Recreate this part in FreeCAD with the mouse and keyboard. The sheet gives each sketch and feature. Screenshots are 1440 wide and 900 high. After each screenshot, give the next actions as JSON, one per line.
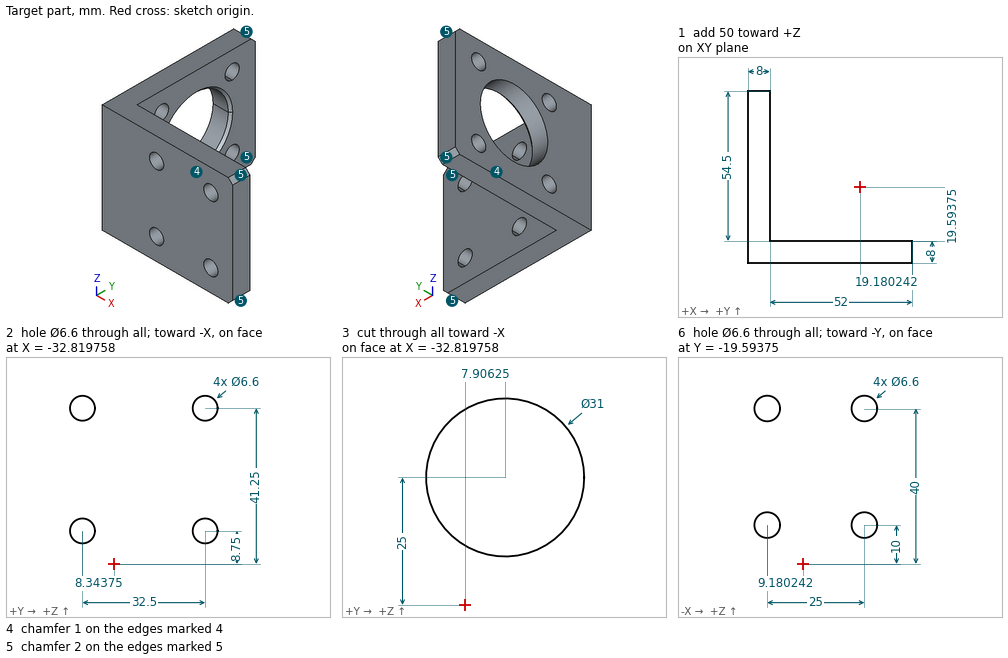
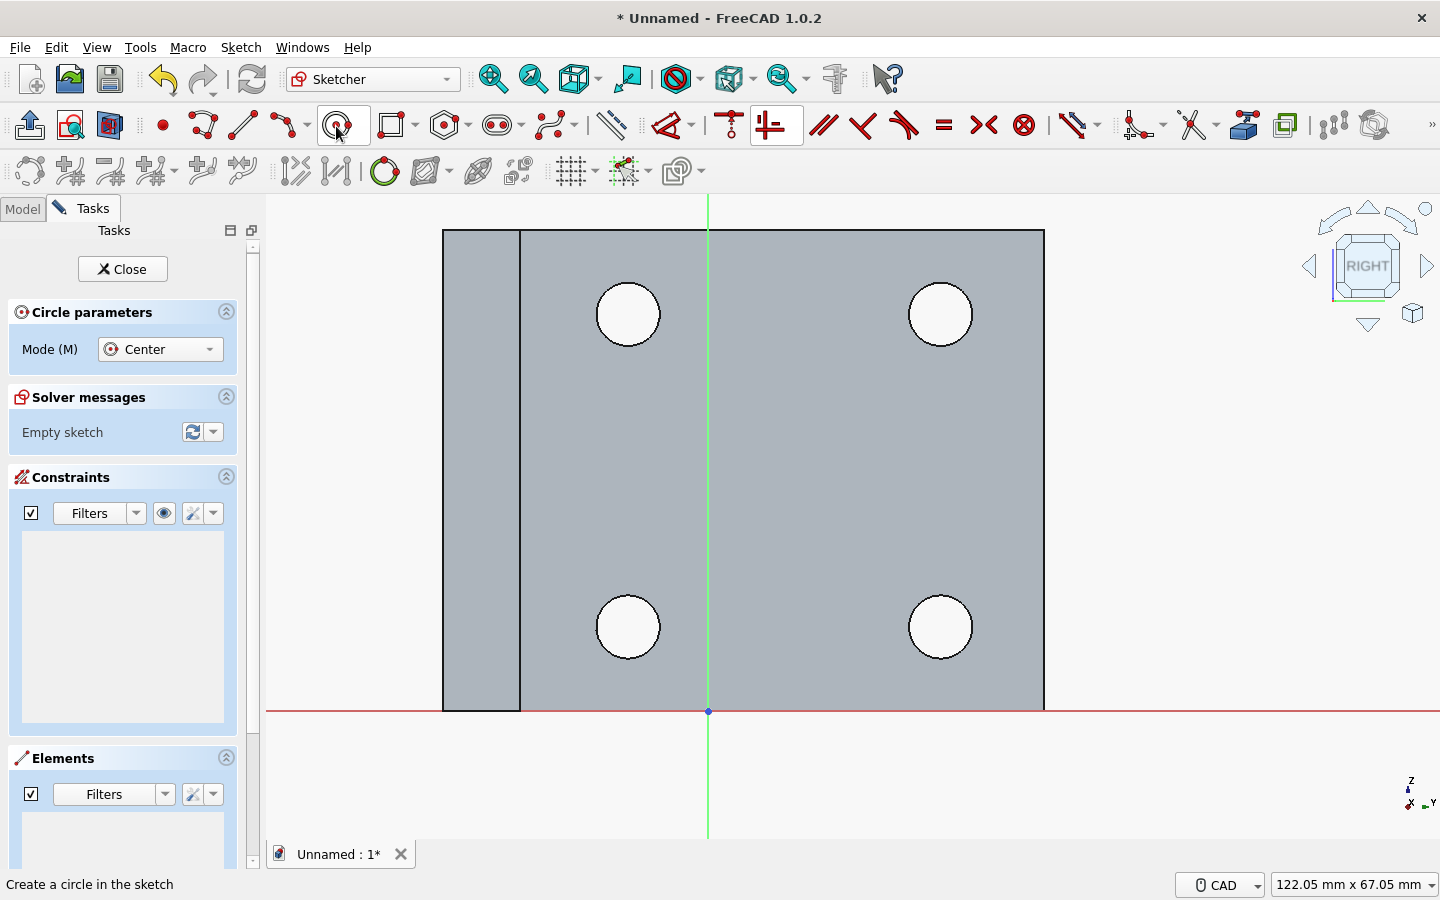
{"action": "left_click", "coordinate": [784, 471]}
{"action": "mouse_move", "coordinate": [890, 365]}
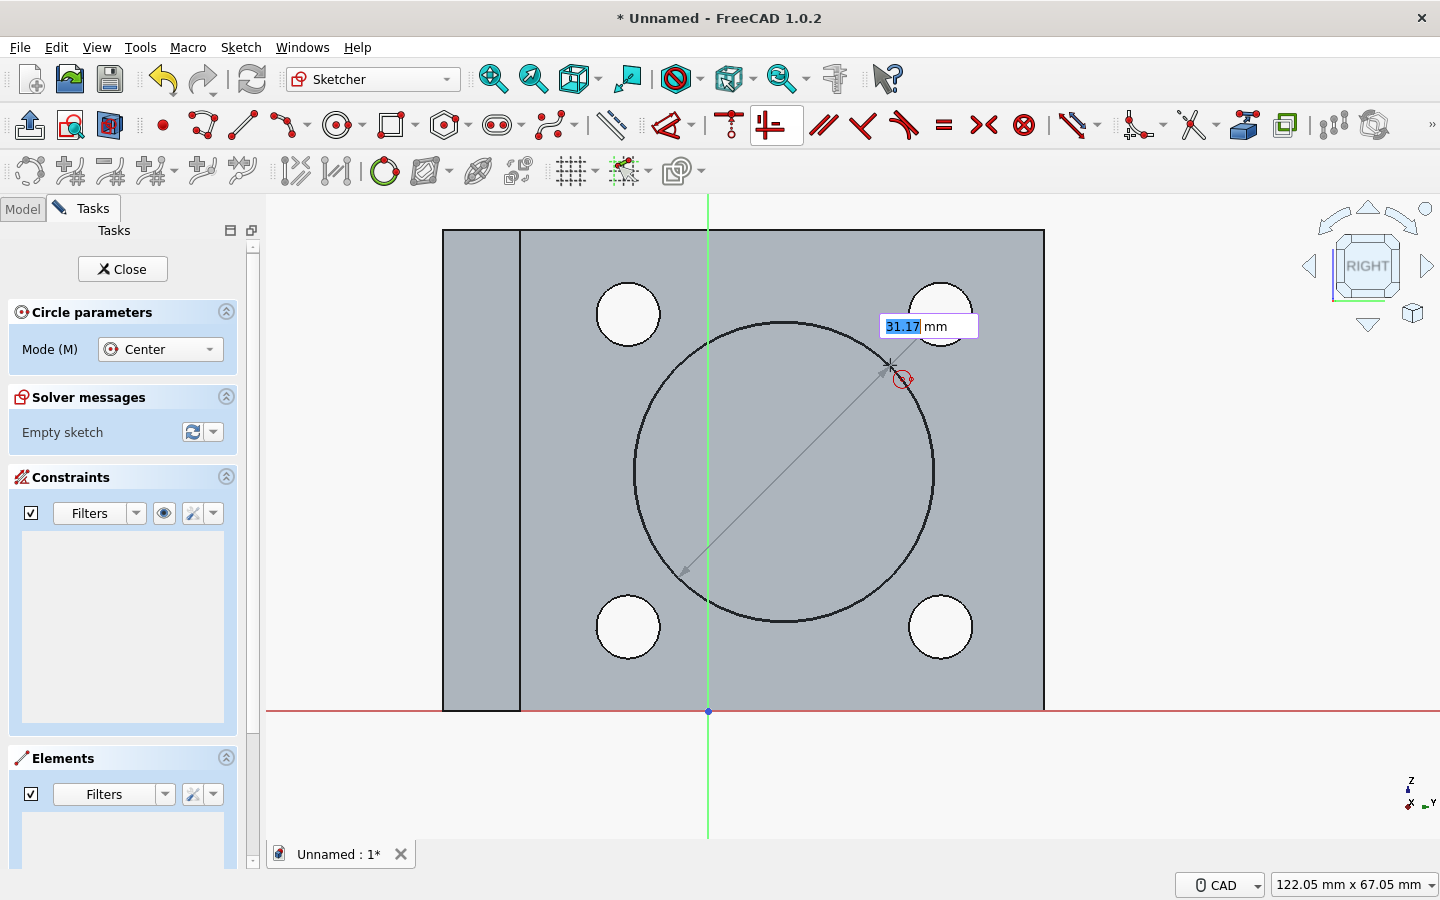
{"action": "type", "text": "31"}
{"action": "key", "text": "Return"}
{"action": "key", "text": "Escape"}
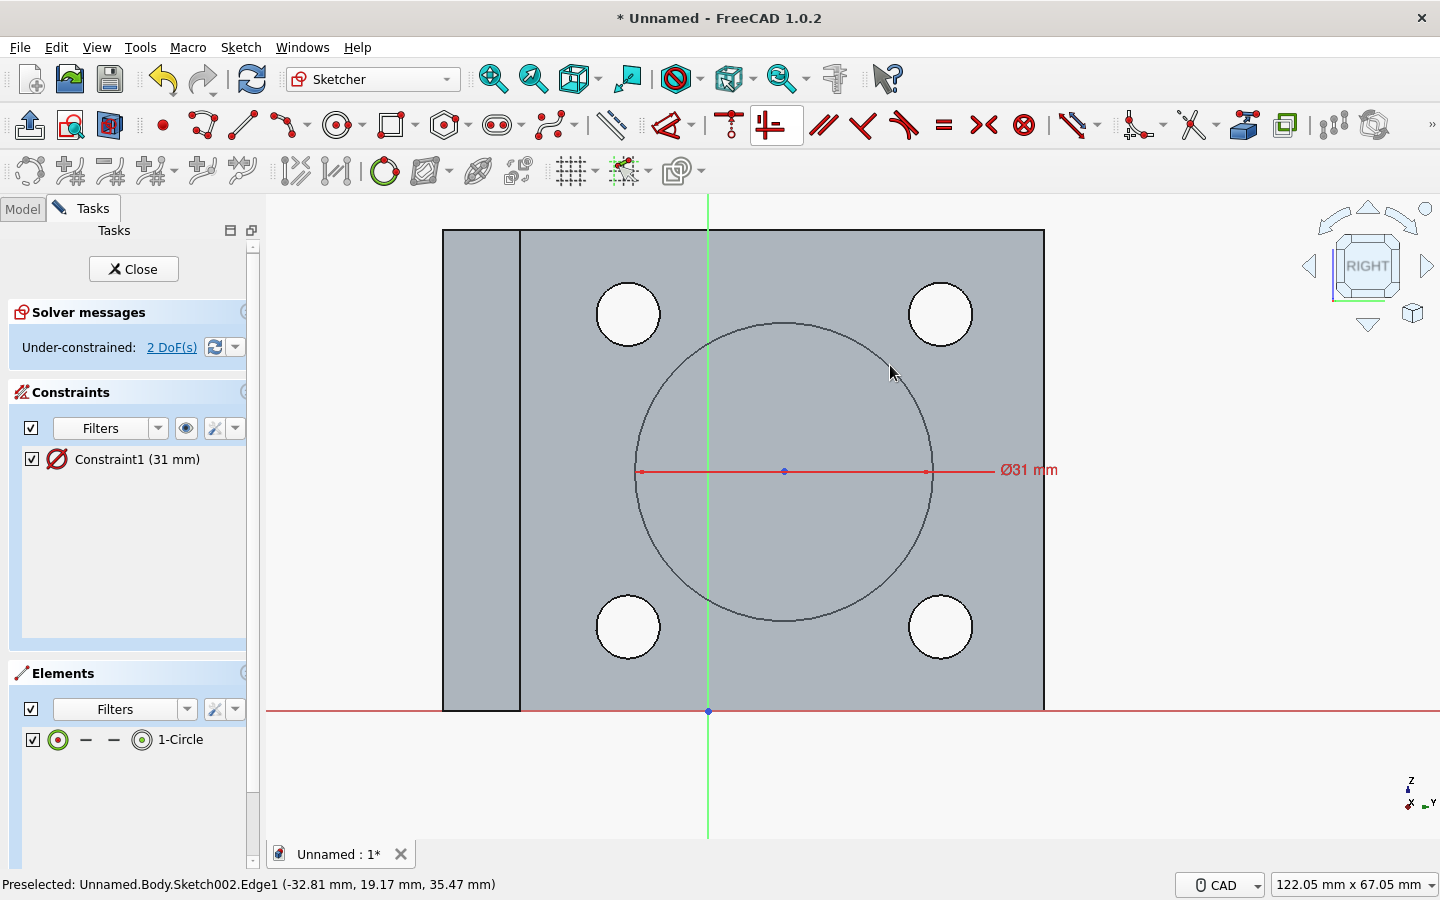
{"action": "left_click", "coordinate": [666, 126]}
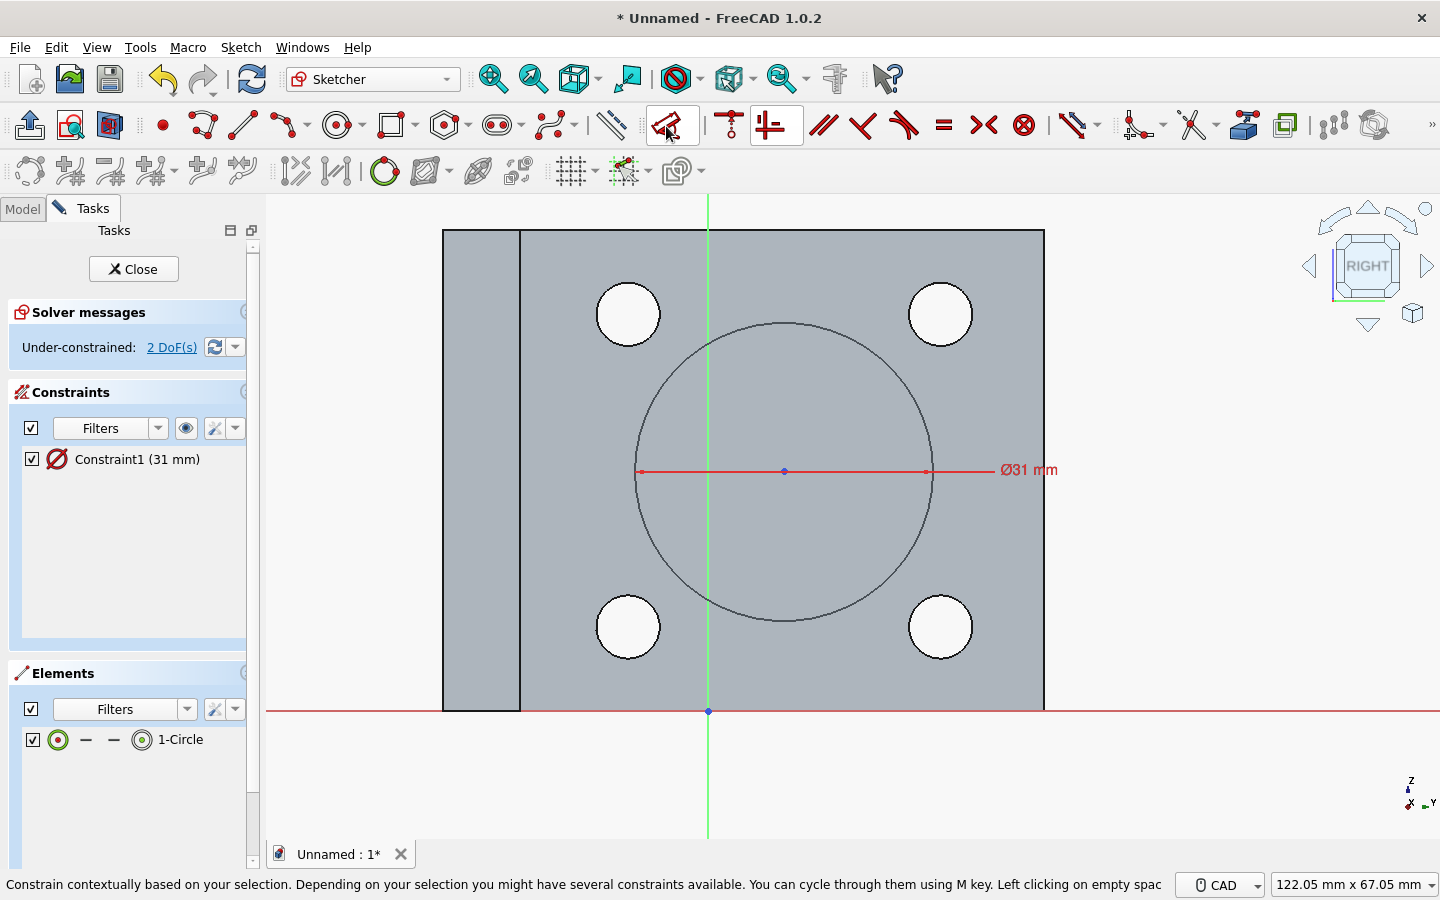
{"action": "left_click", "coordinate": [784, 472]}
{"action": "left_click", "coordinate": [674, 592]}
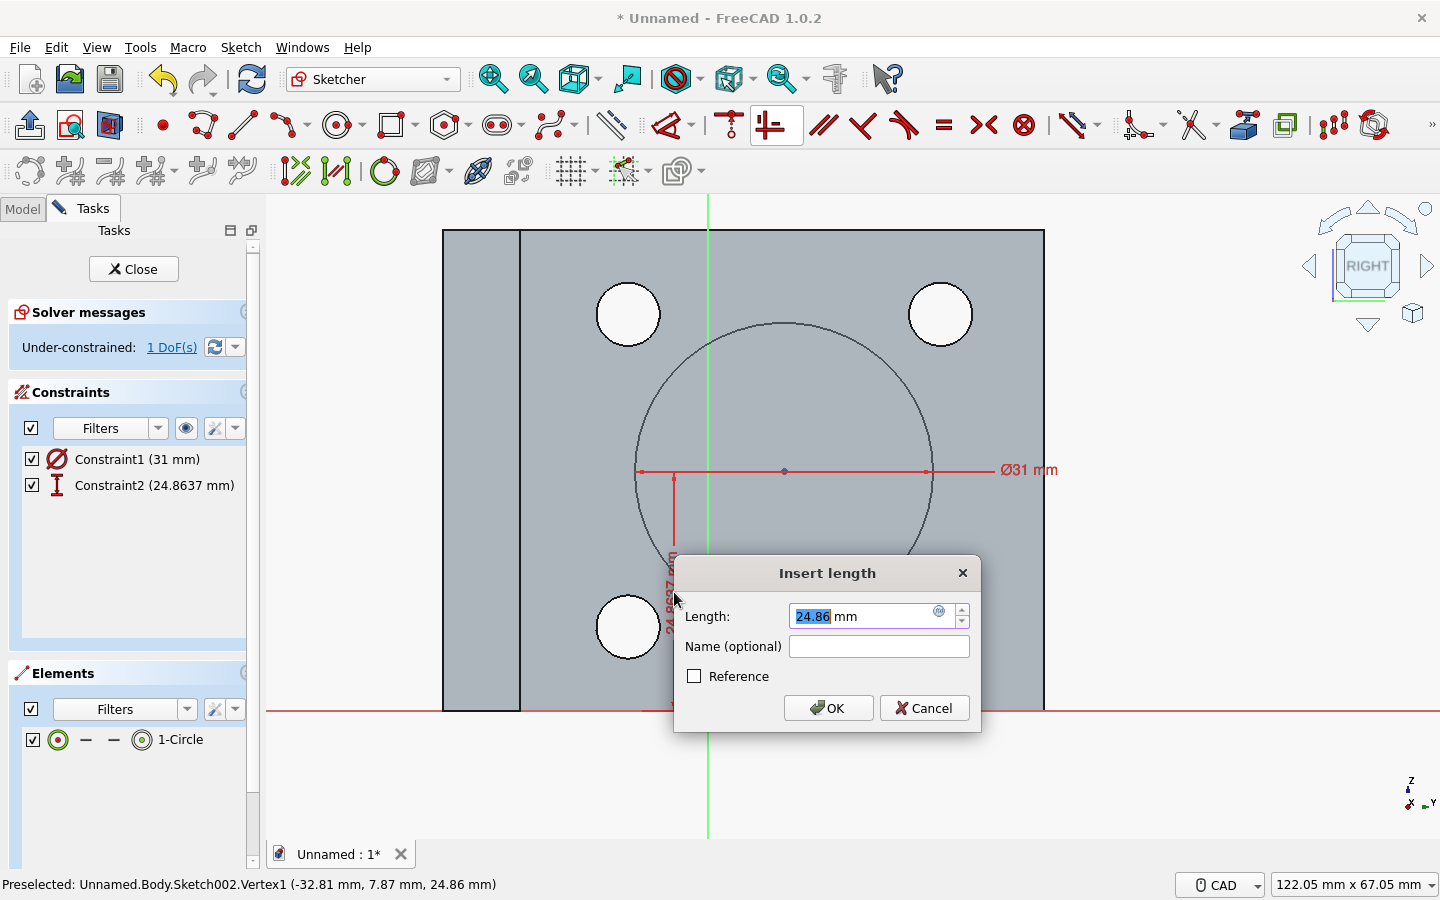
{"action": "type", "text": "25"}
{"action": "key", "text": "Return"}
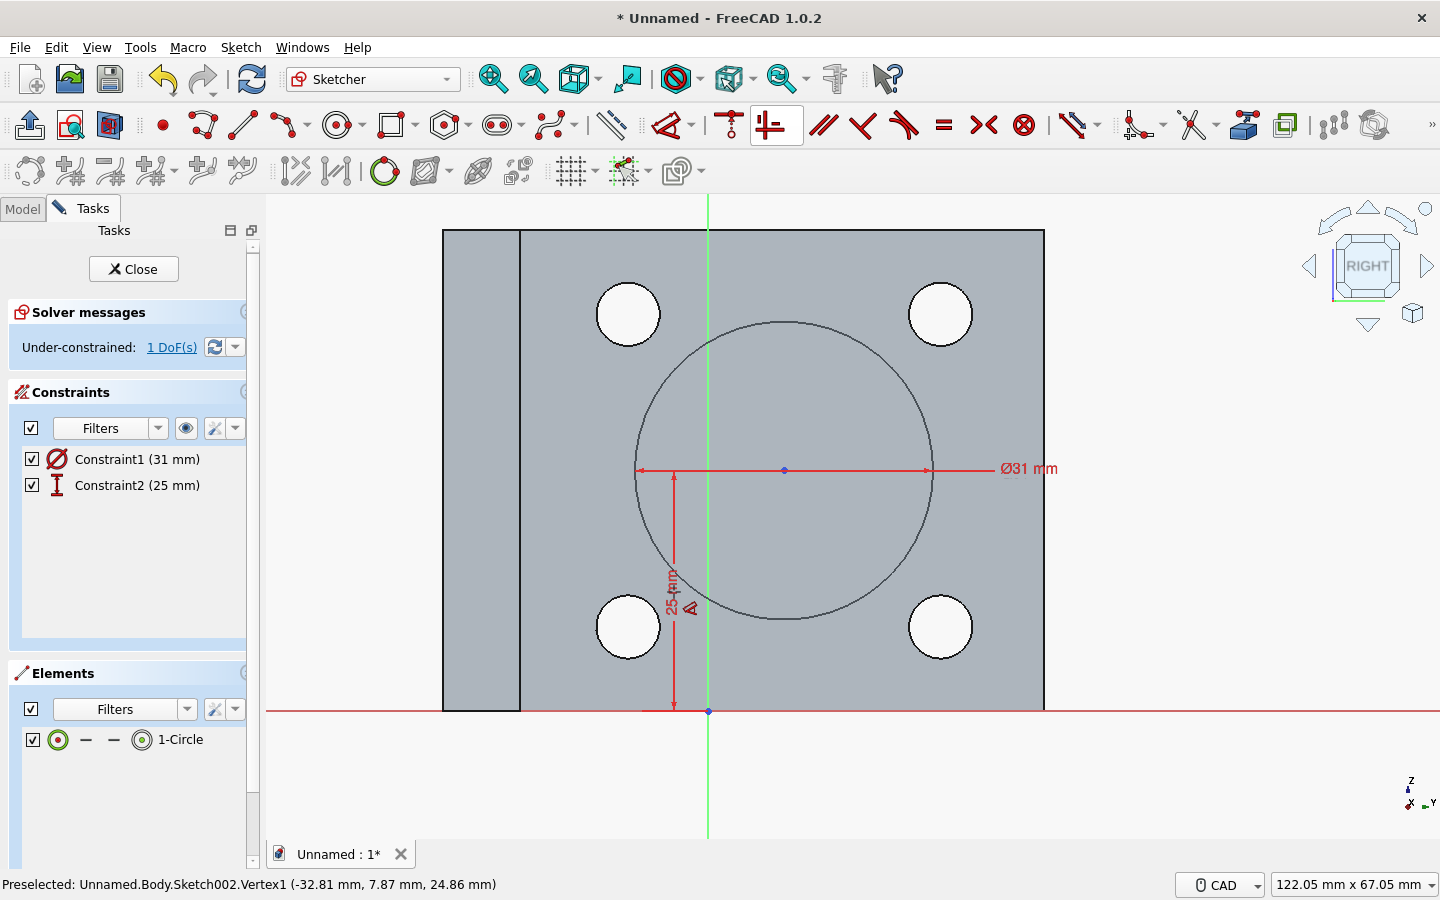
{"action": "left_click", "coordinate": [784, 471]}
{"action": "left_click", "coordinate": [746, 745]}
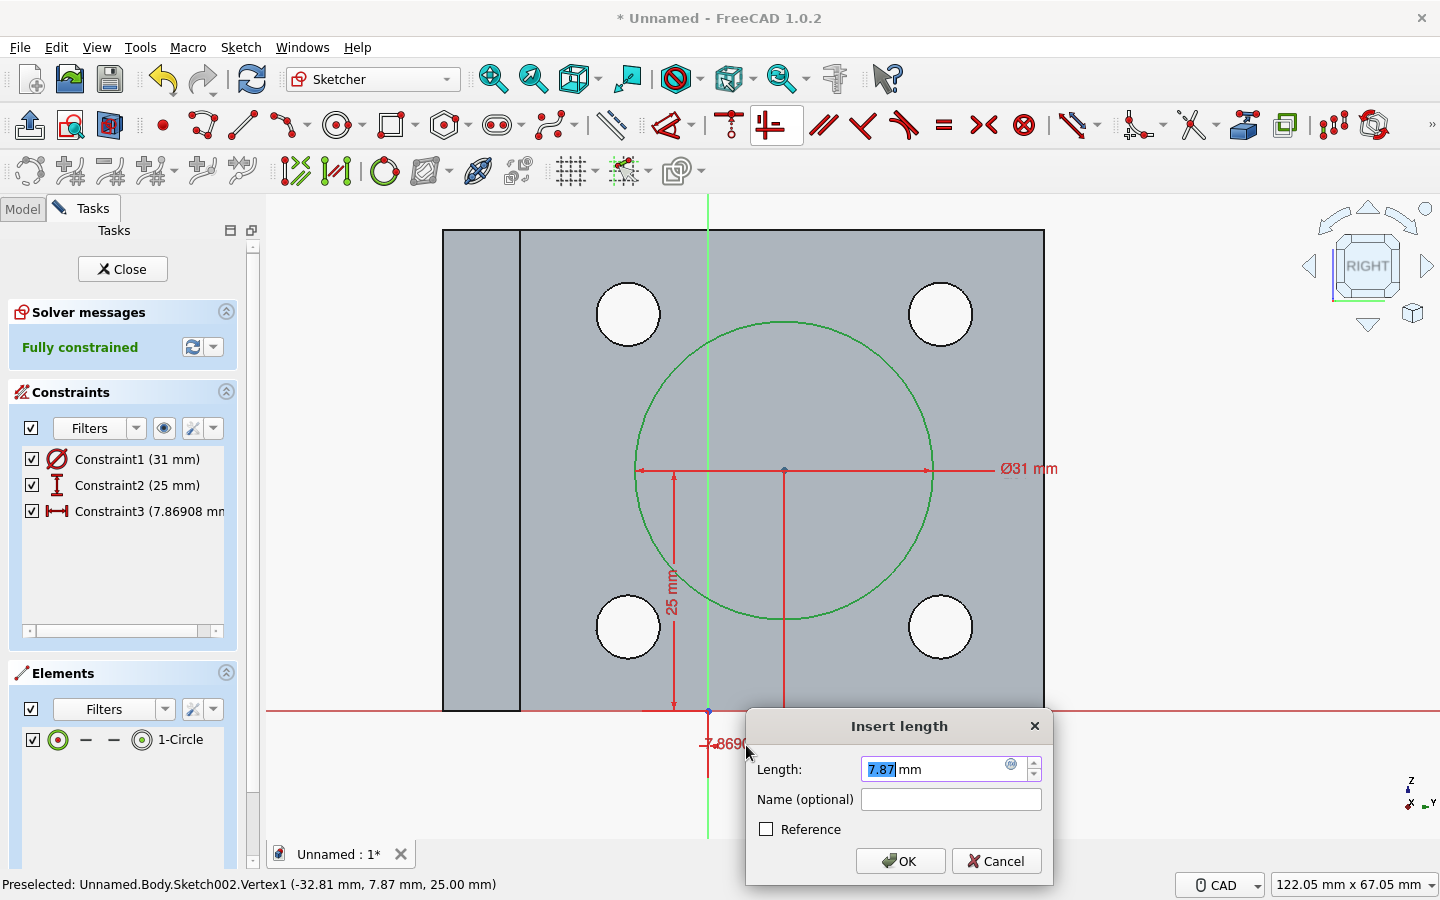
{"action": "type", "text": "7.90625"}
{"action": "key", "text": "Return"}
{"action": "key", "text": "Escape"}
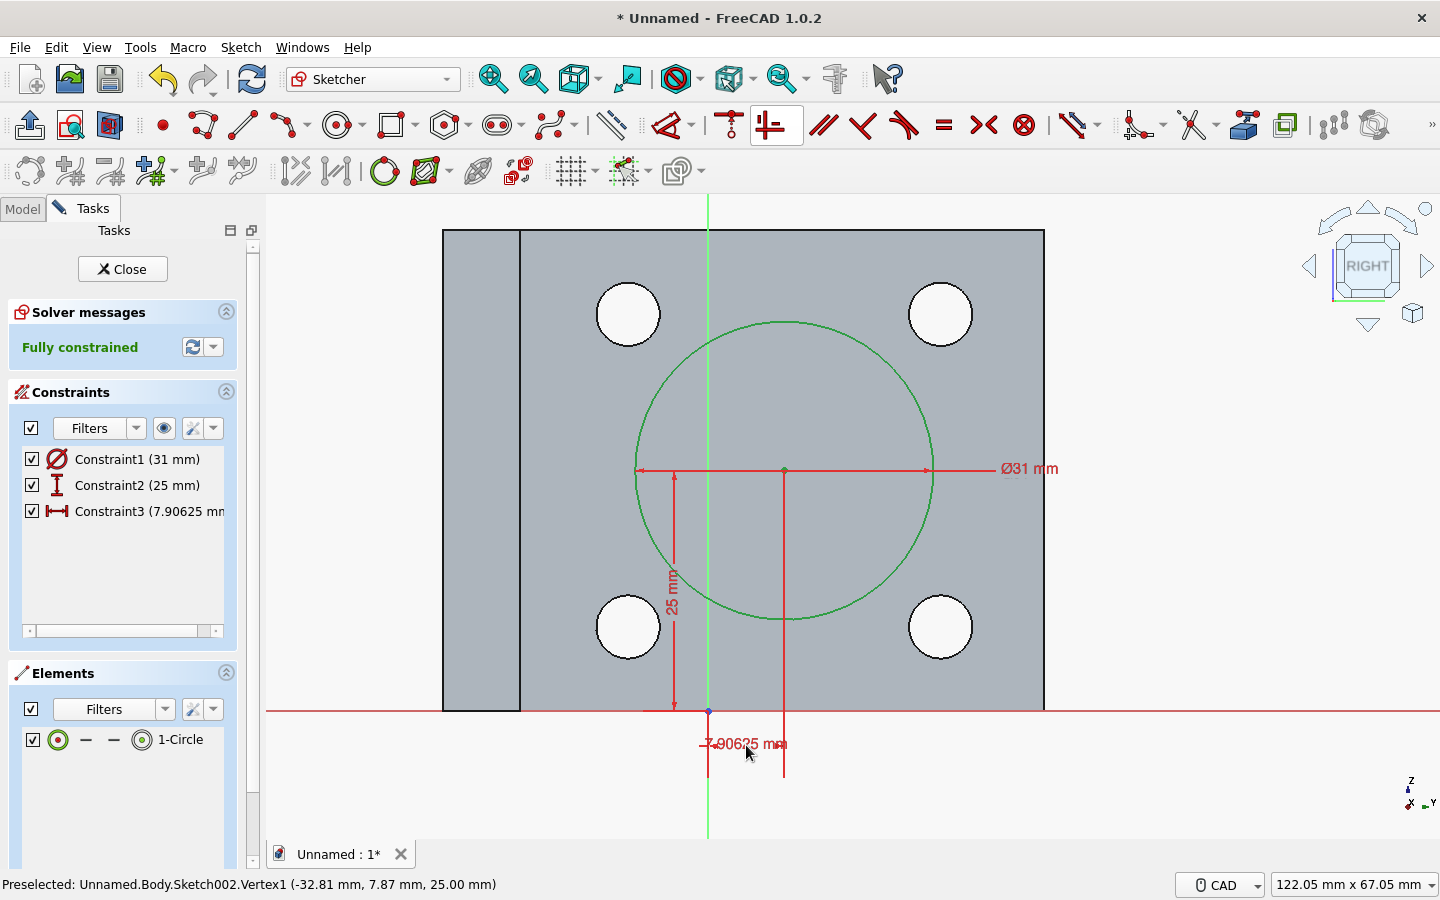
{"action": "left_click", "coordinate": [123, 269]}